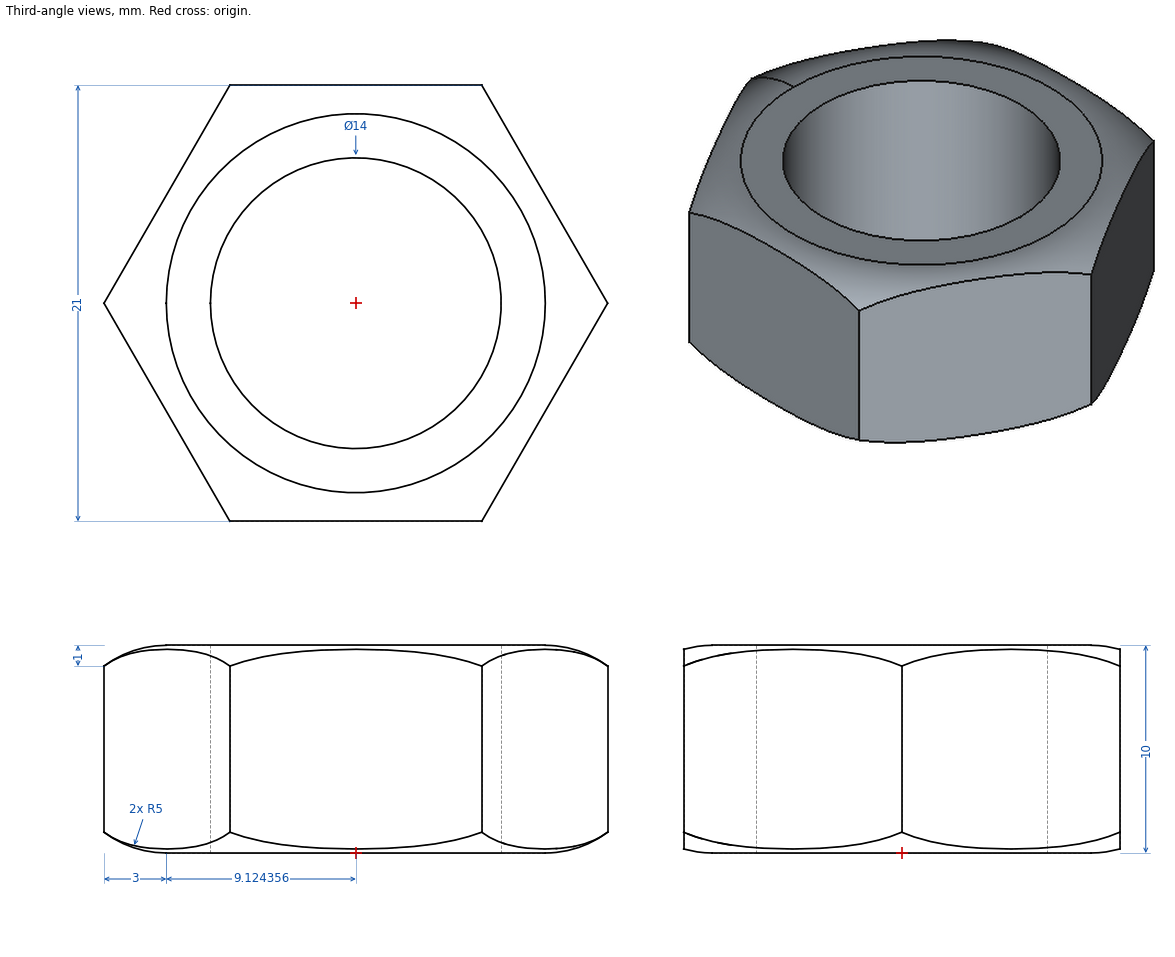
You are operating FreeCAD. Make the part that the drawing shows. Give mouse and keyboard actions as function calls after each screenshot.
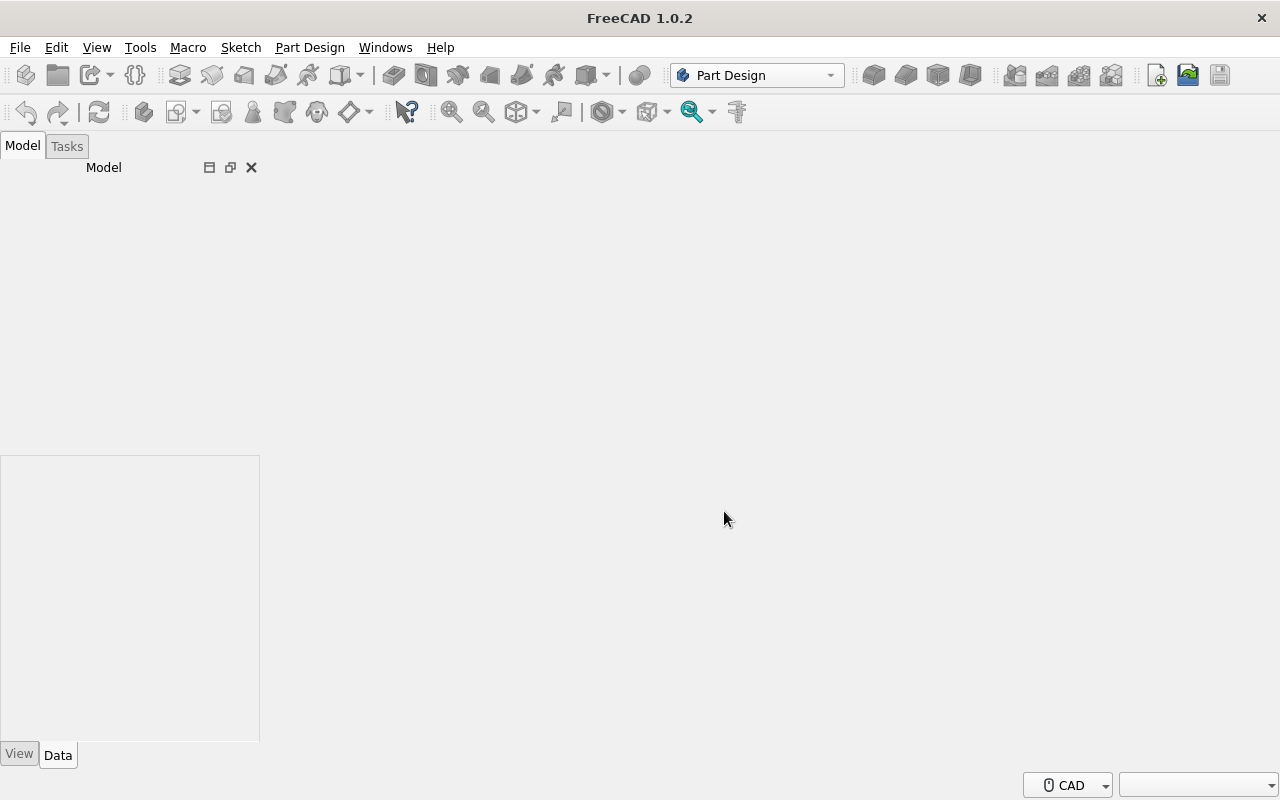
key(ctrl+n)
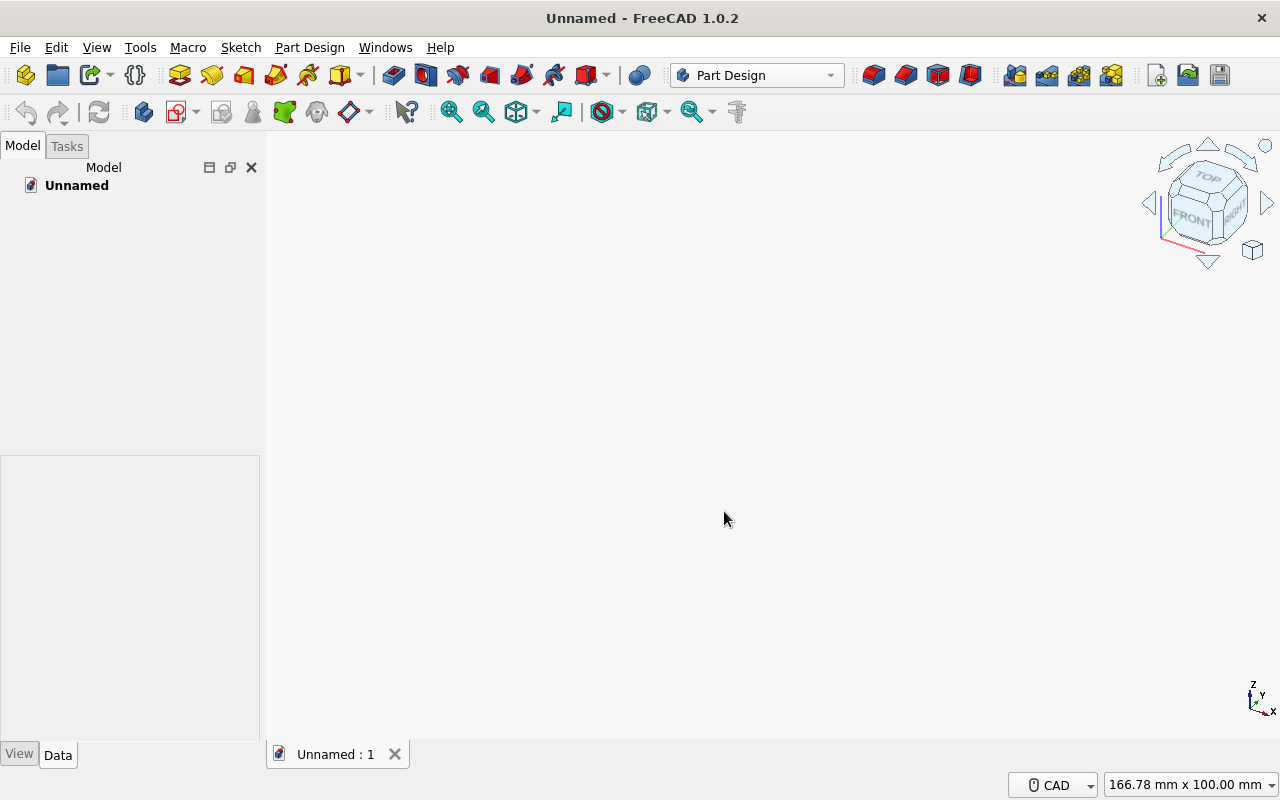
click(176, 112)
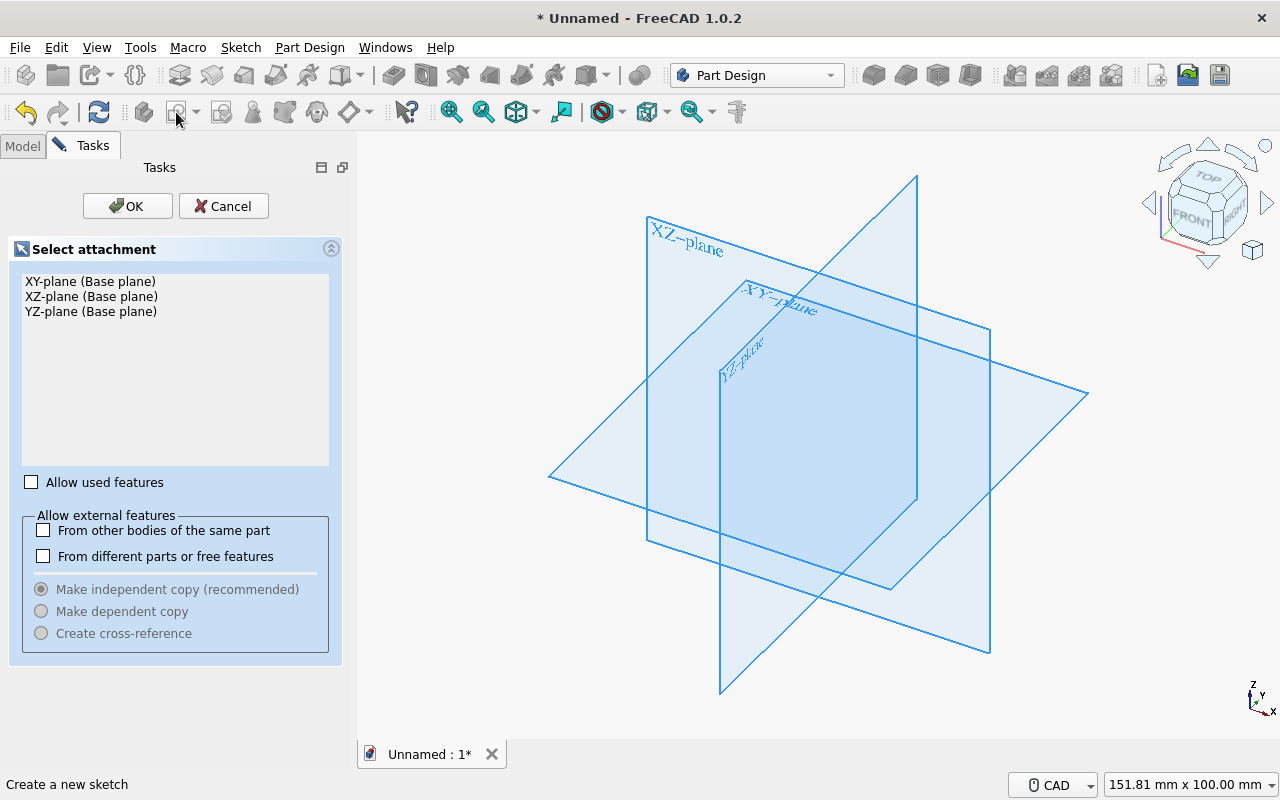
click(82, 282)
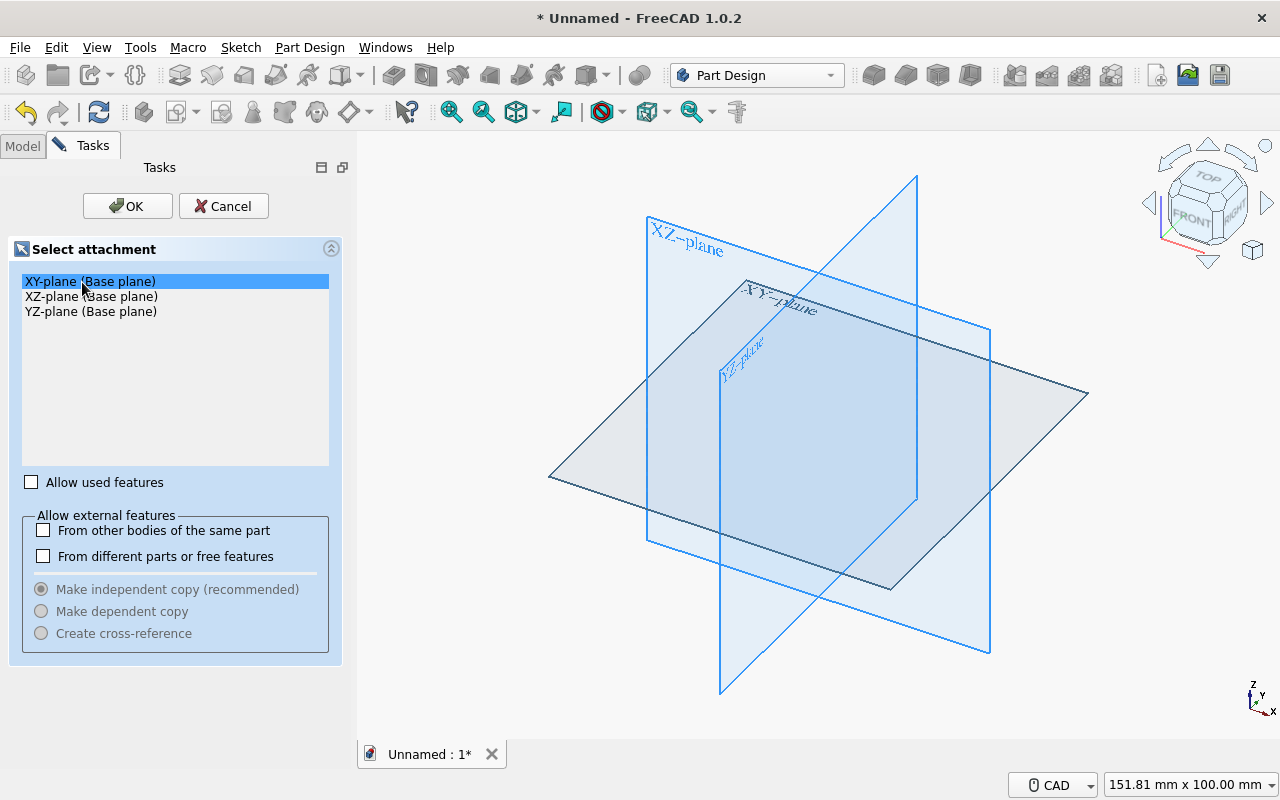
click(128, 206)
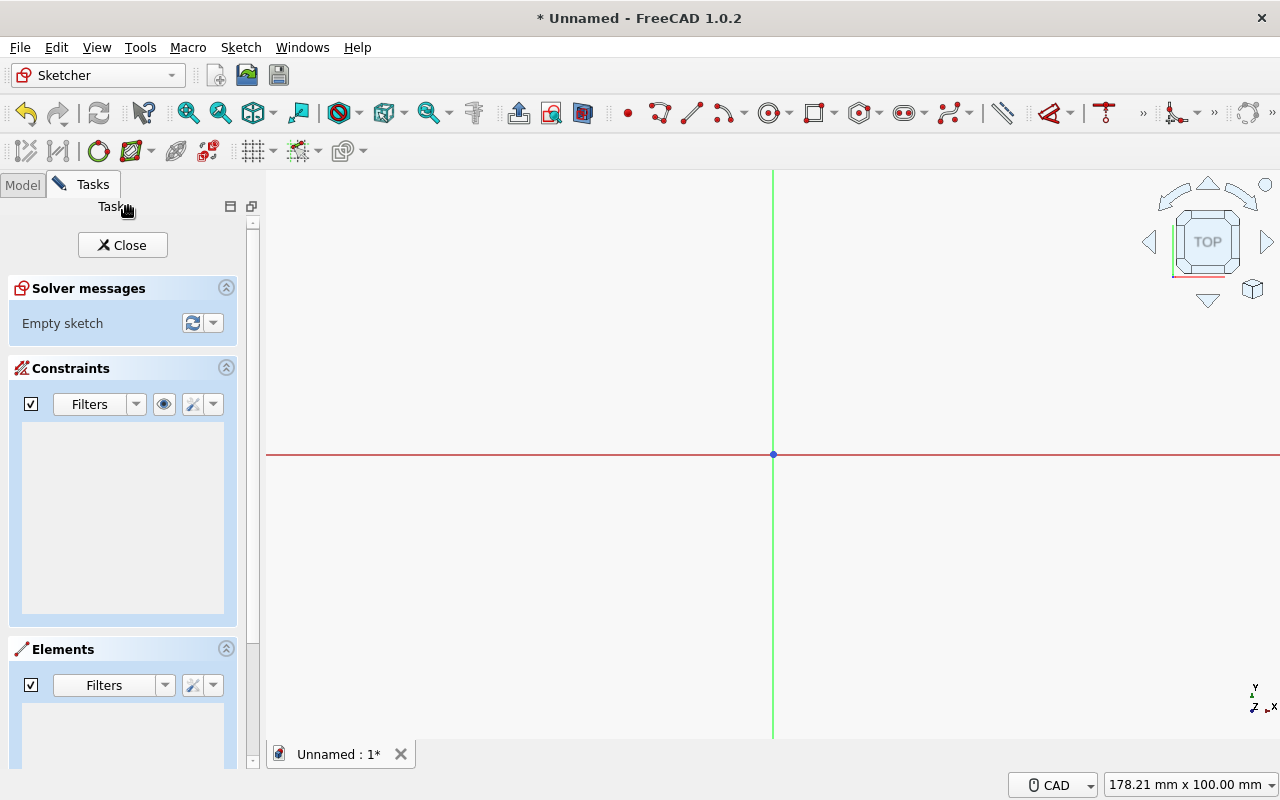
scroll(803, 455, up, 6)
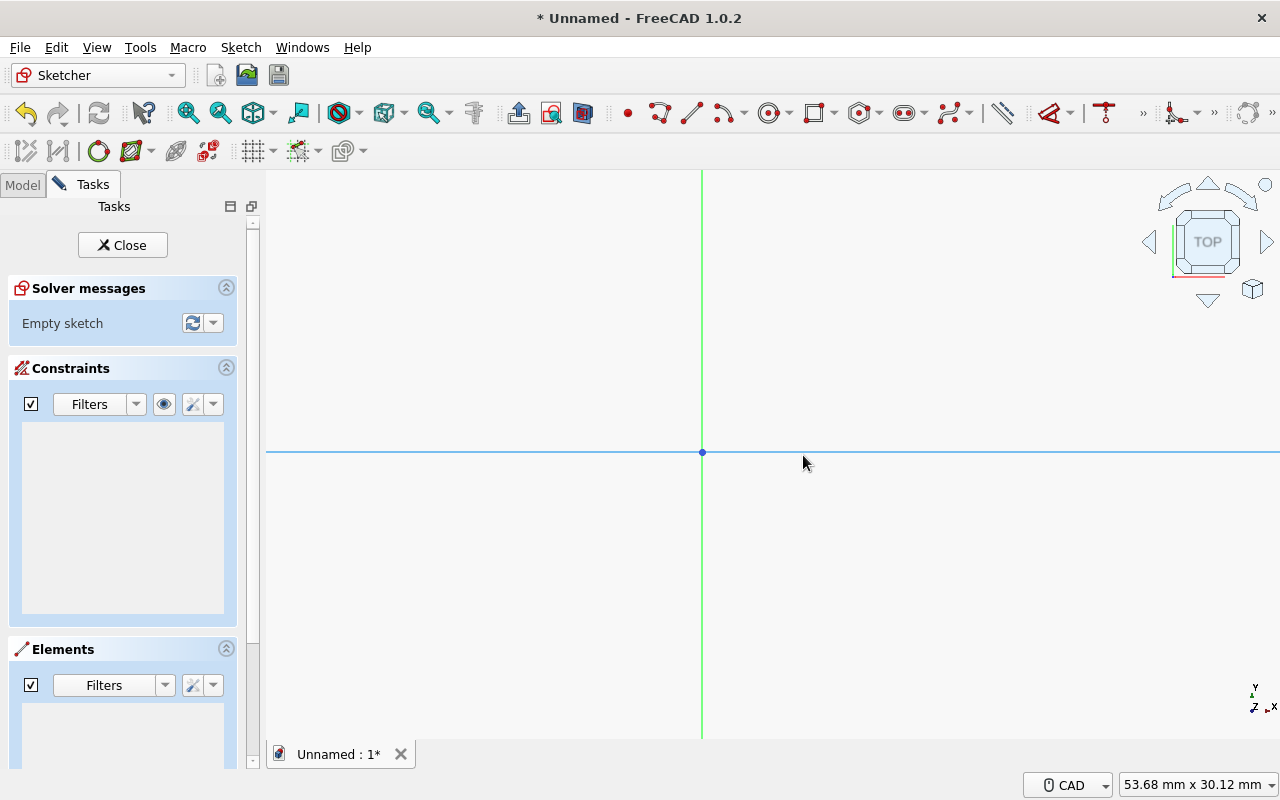
click(860, 114)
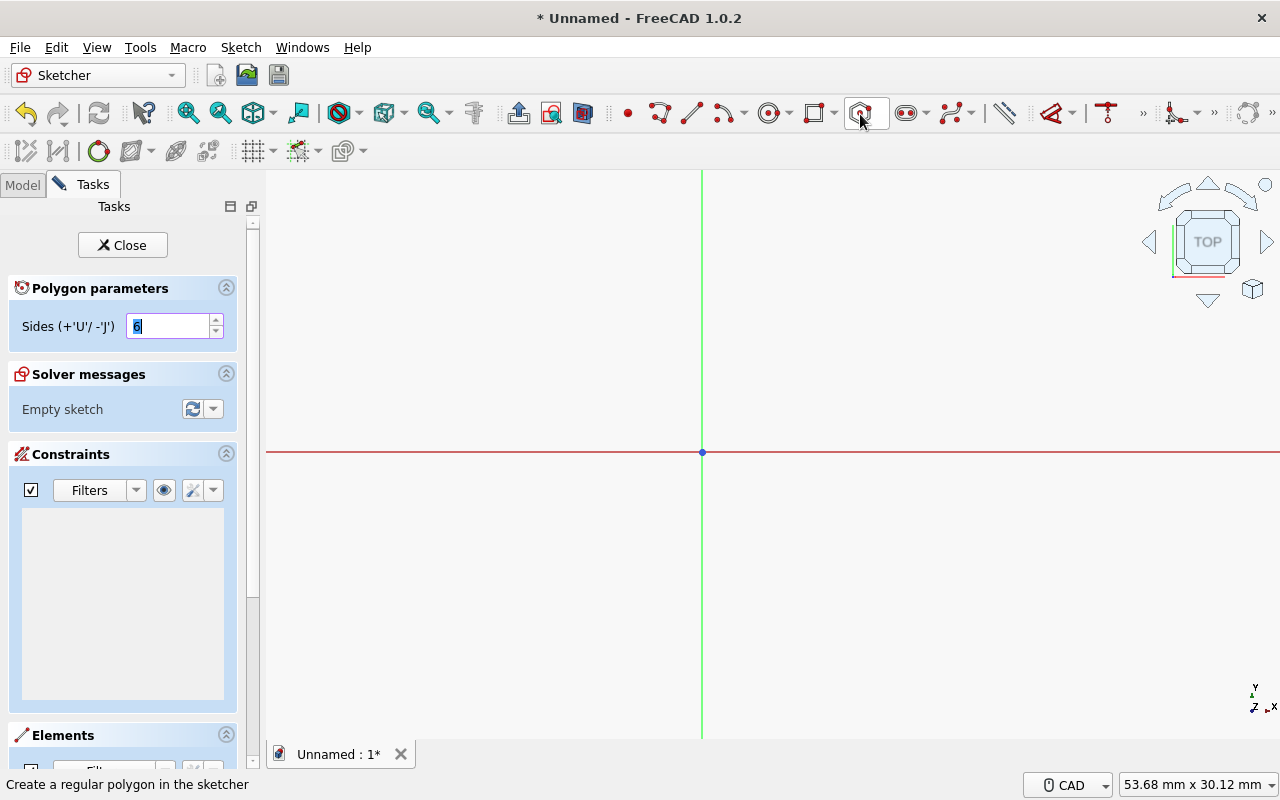
click(702, 452)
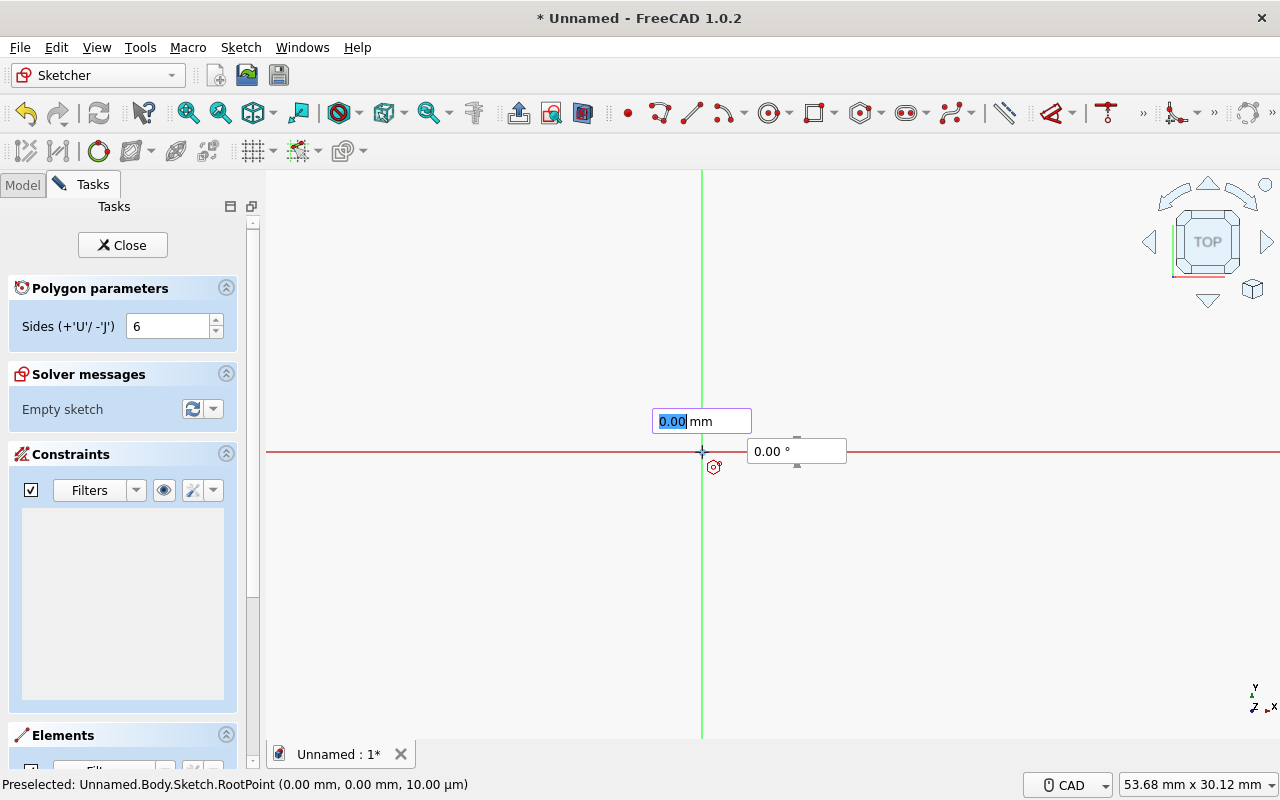
click(931, 452)
right_click(931, 452)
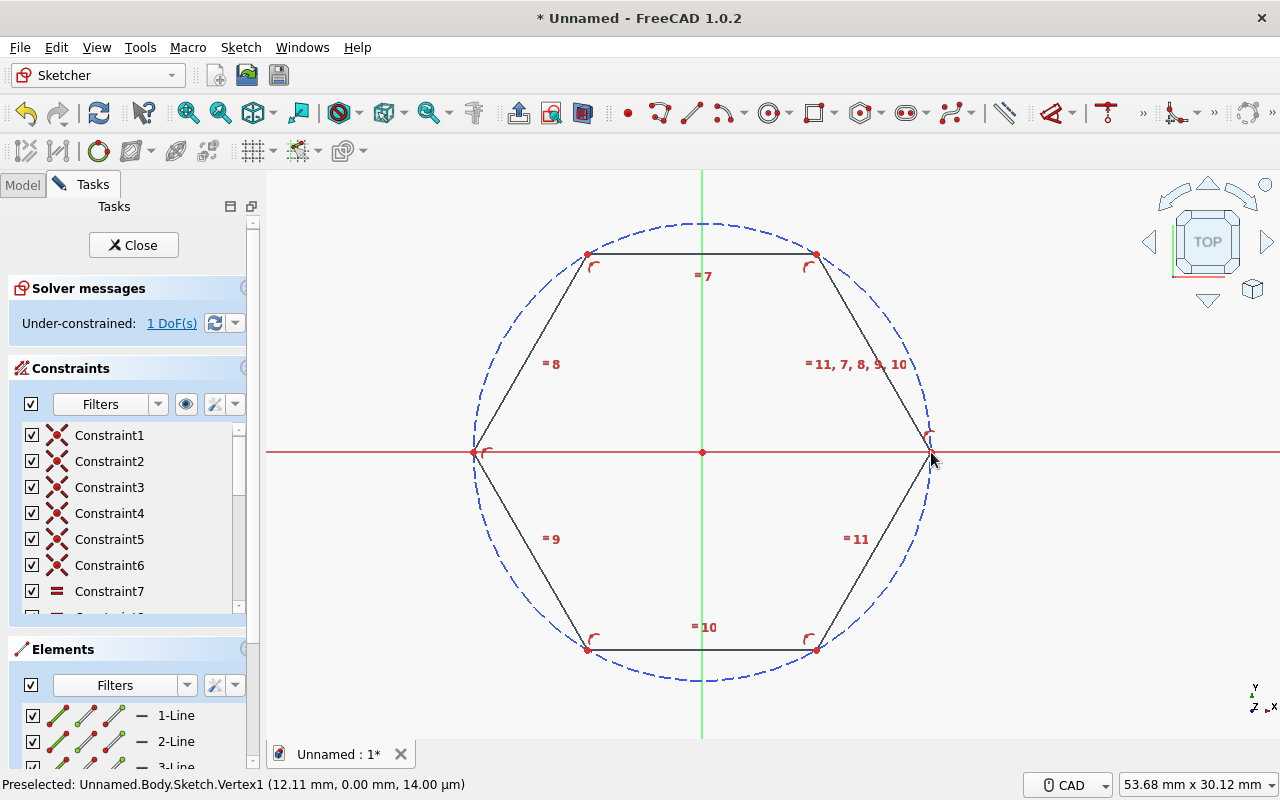
click(588, 650)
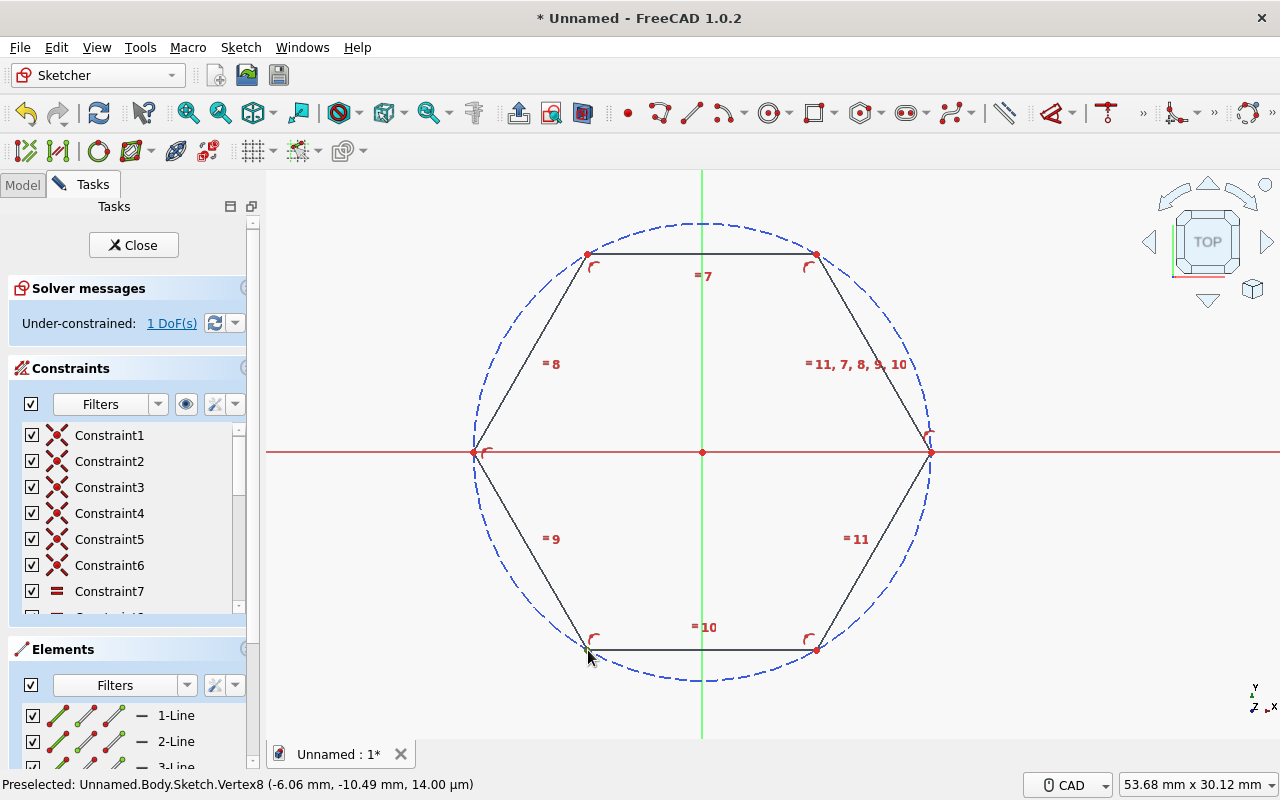
click(817, 254)